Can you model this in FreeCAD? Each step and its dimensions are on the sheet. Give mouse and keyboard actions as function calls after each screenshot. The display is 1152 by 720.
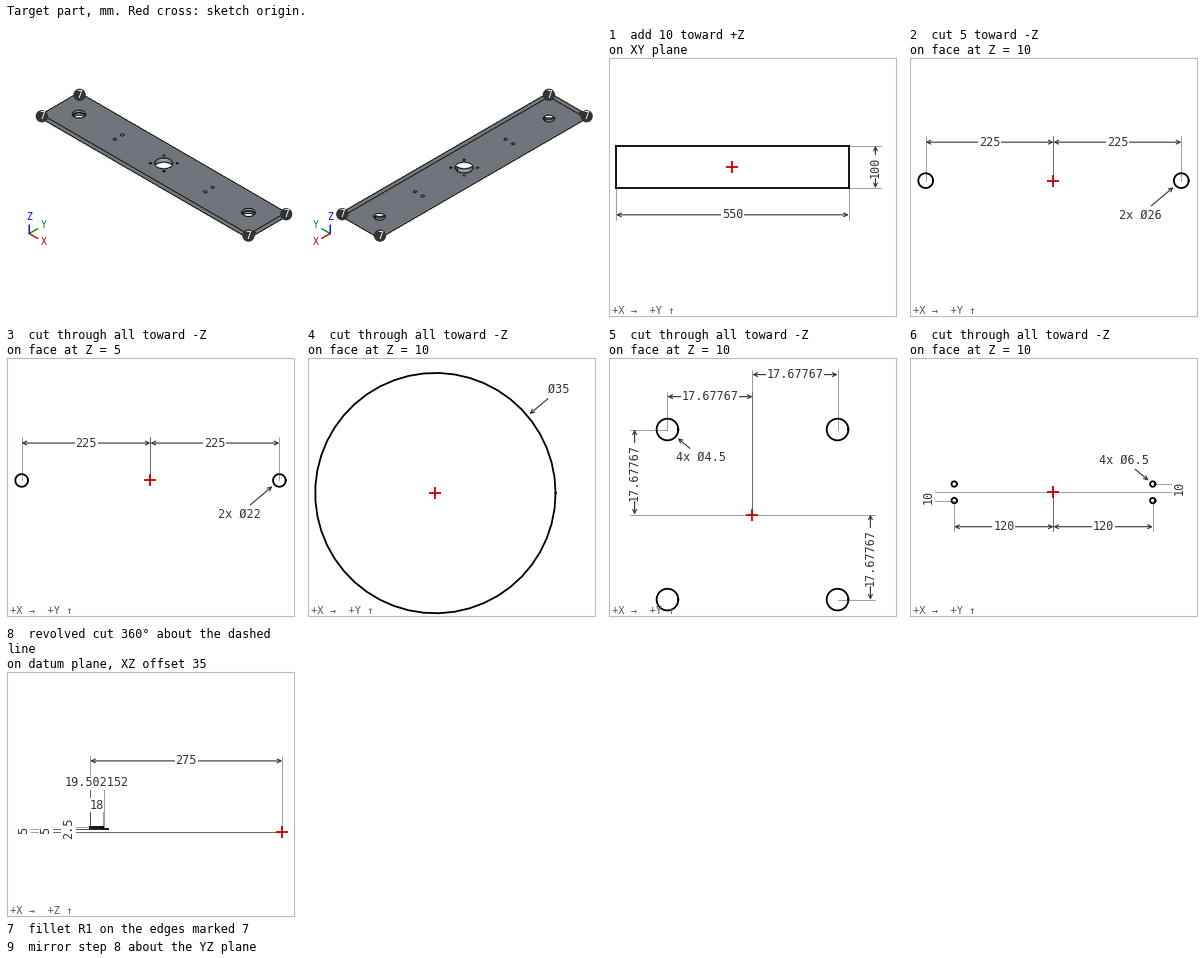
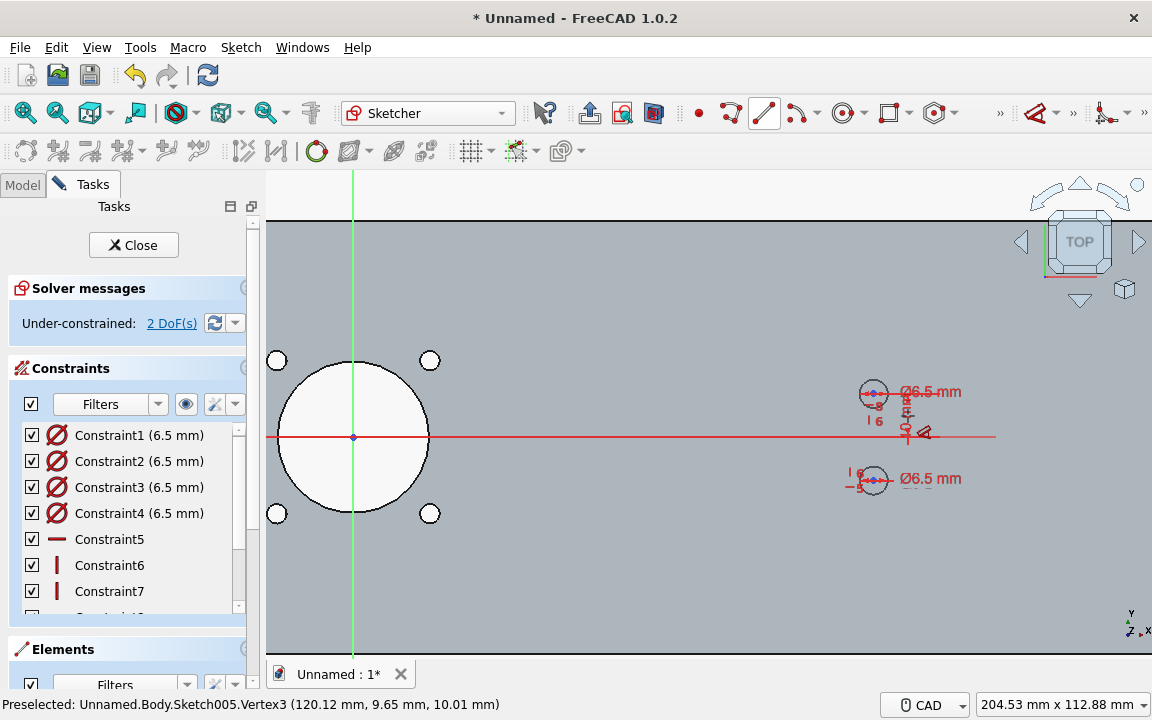
scroll(875, 396, down, 4)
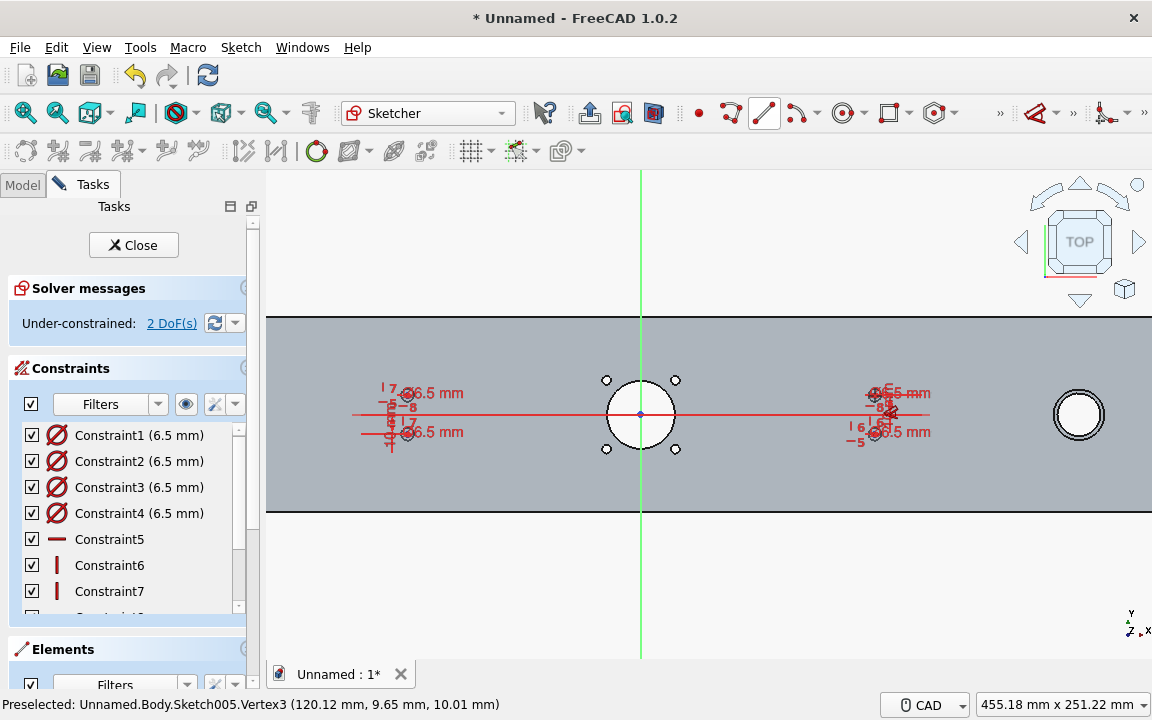
click(408, 434)
click(524, 468)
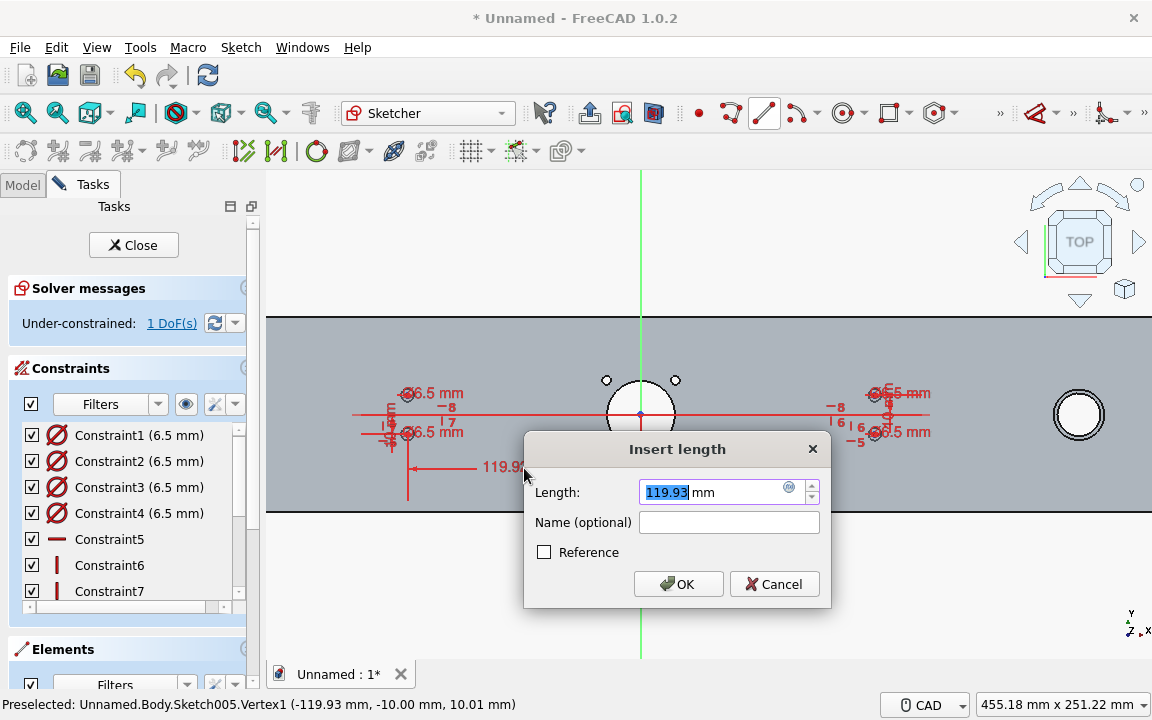
text(120)
key(Return)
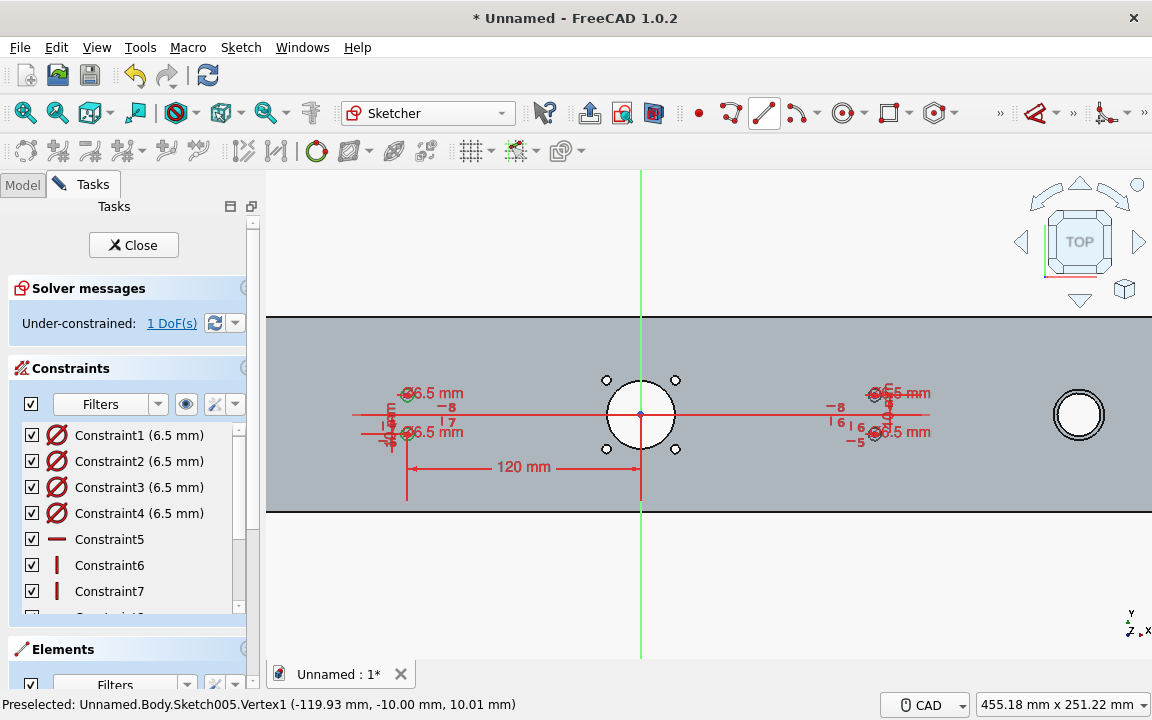
click(875, 434)
click(758, 468)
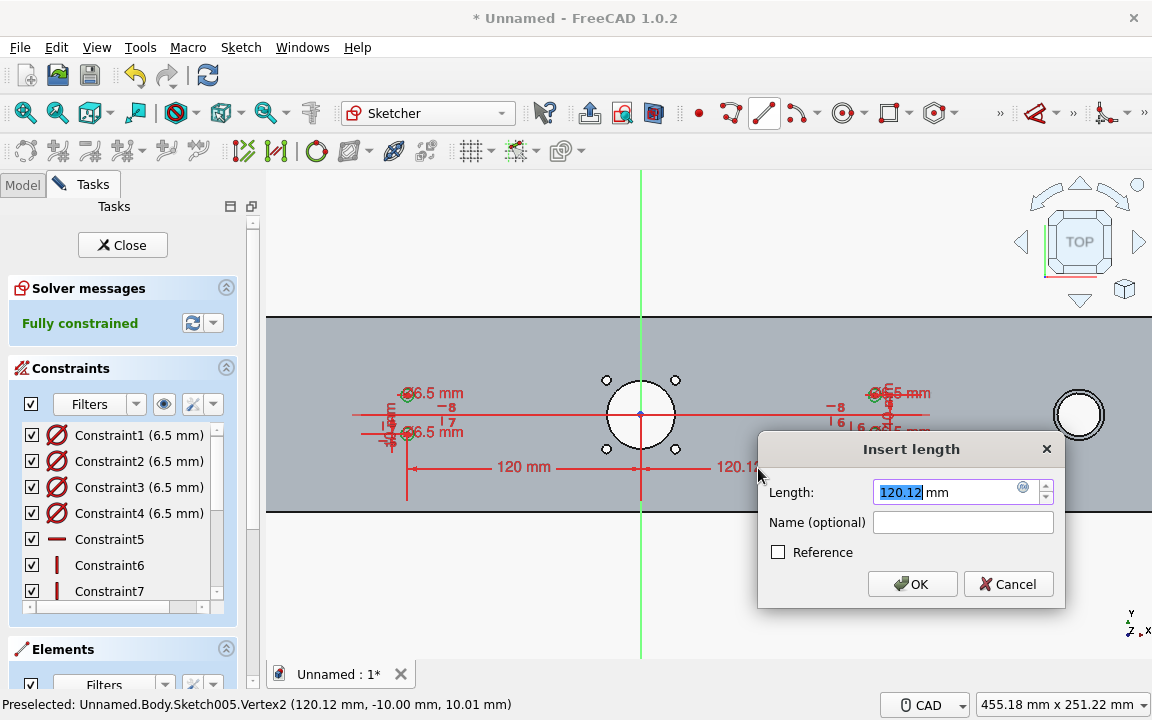
text(120)
key(Return)
key(Escape)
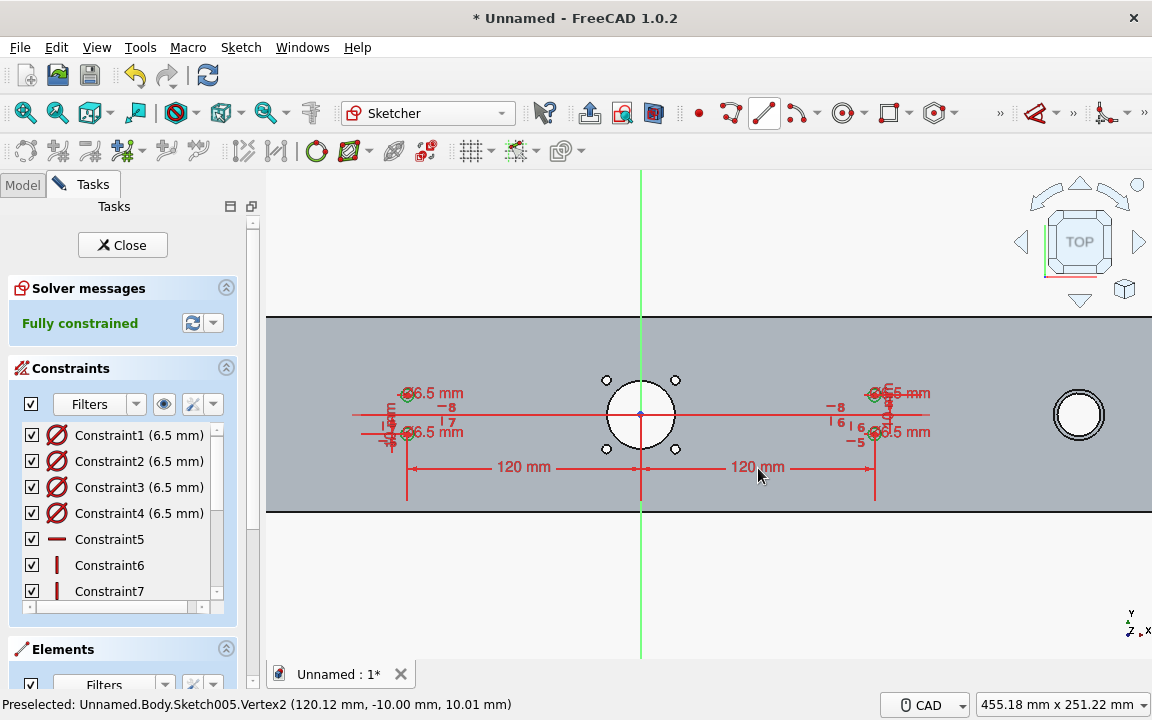
click(123, 245)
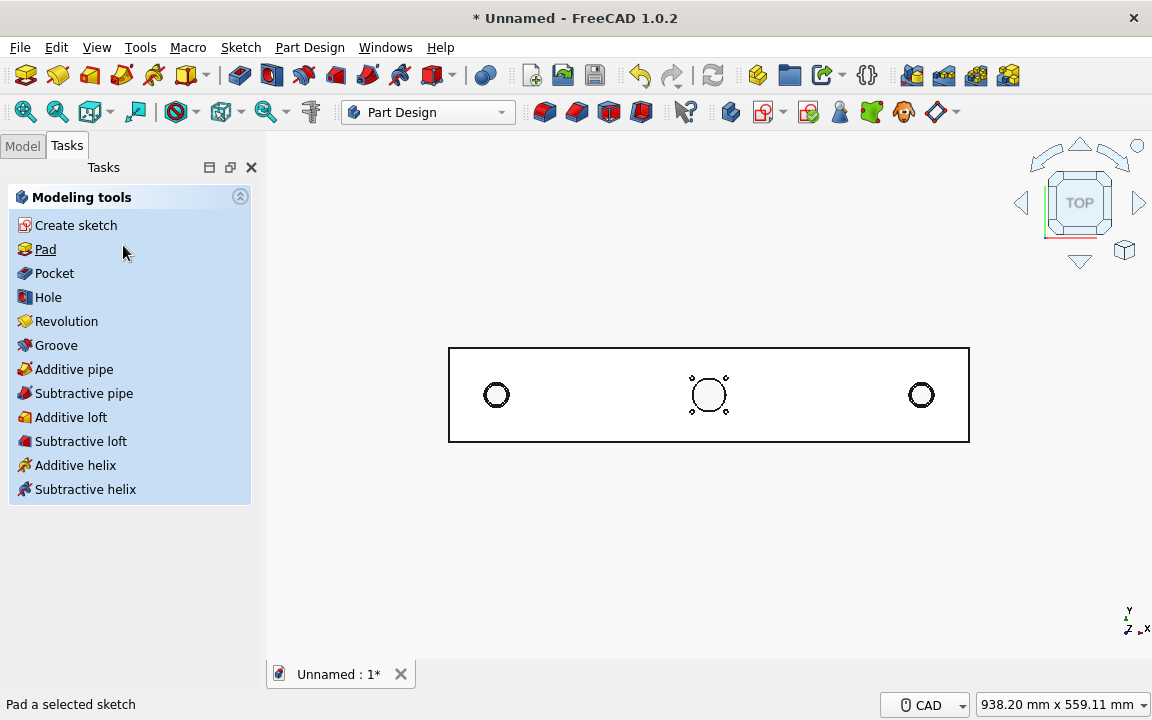
click(240, 76)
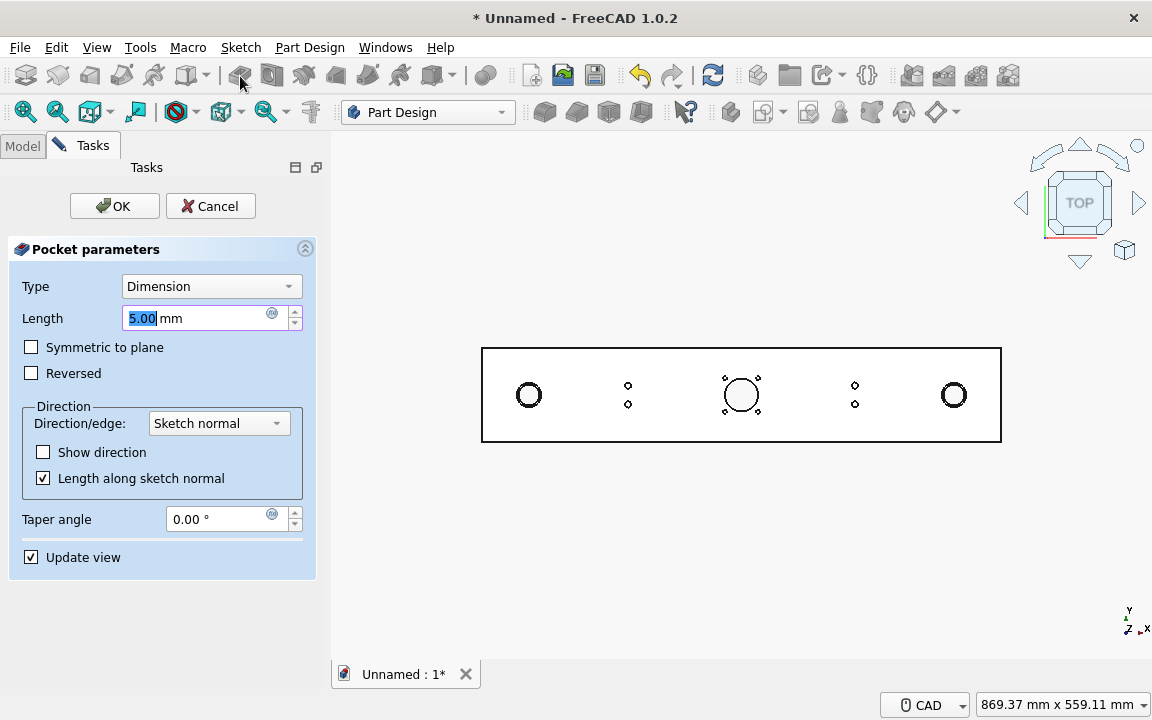
click(212, 286)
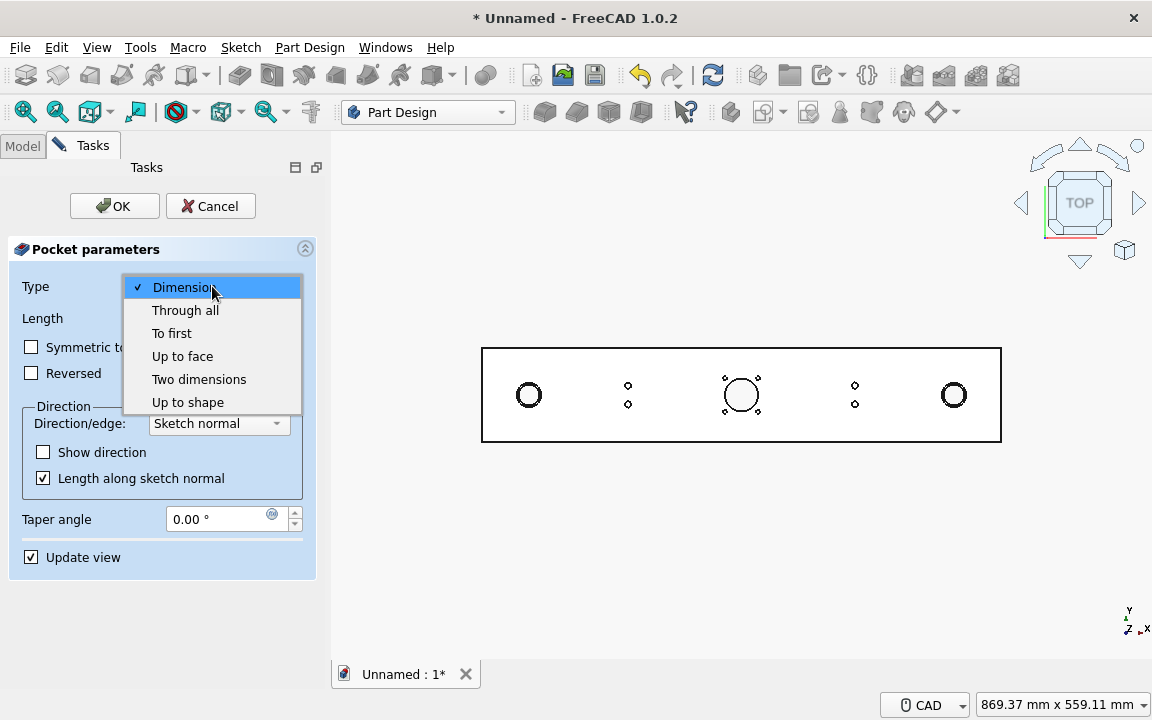
click(212, 310)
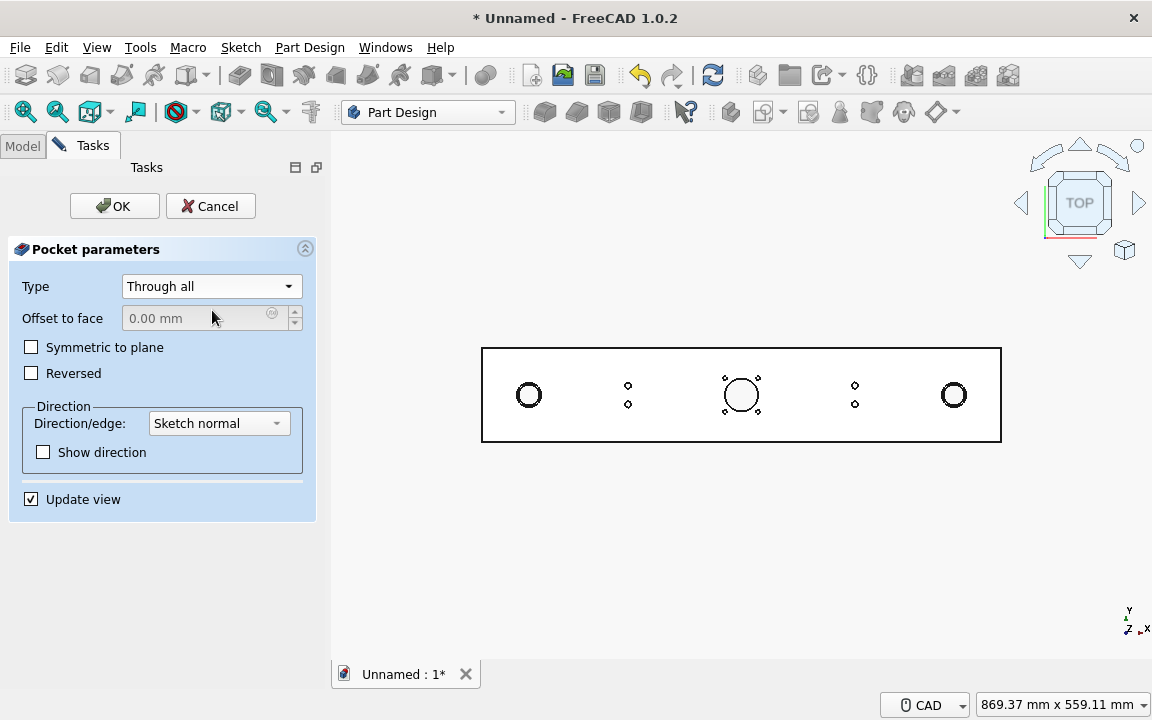
click(115, 206)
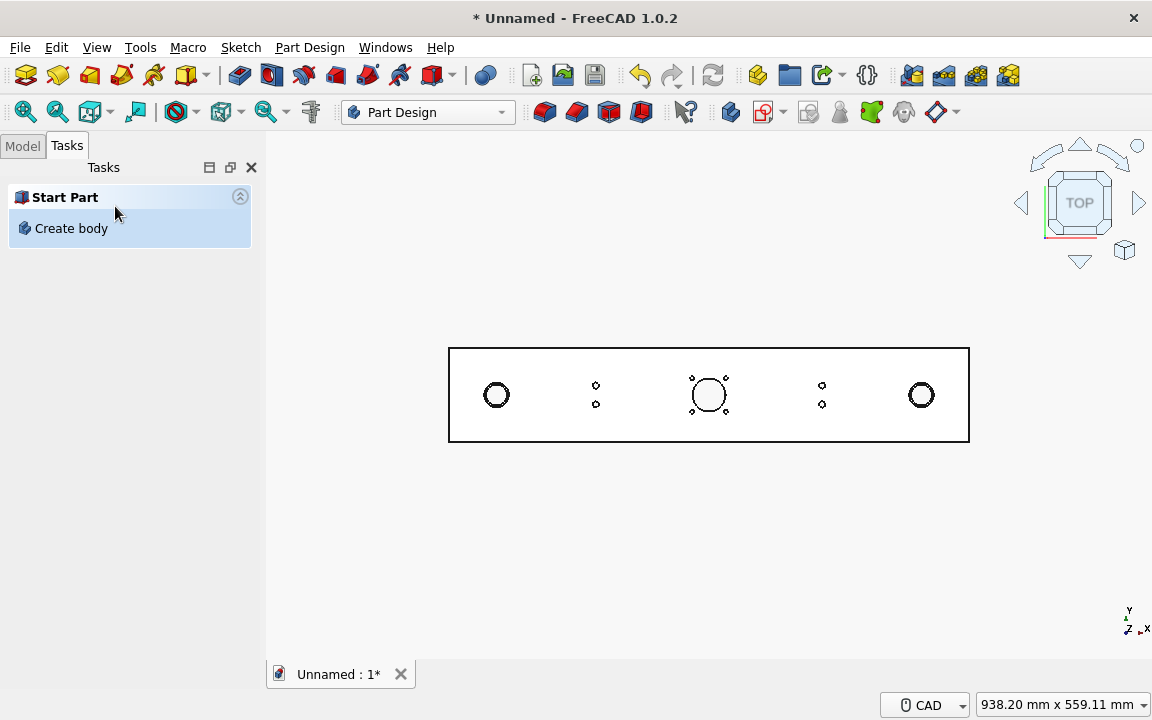
scroll(449, 347, up, 8)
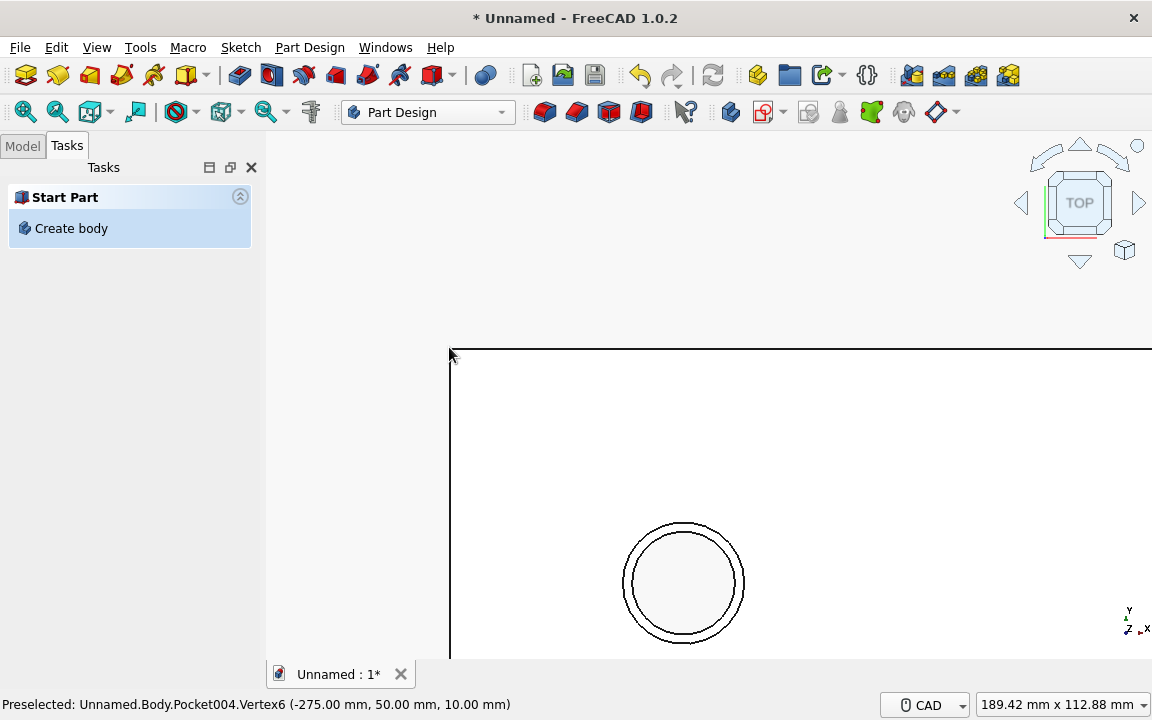
click(26, 112)